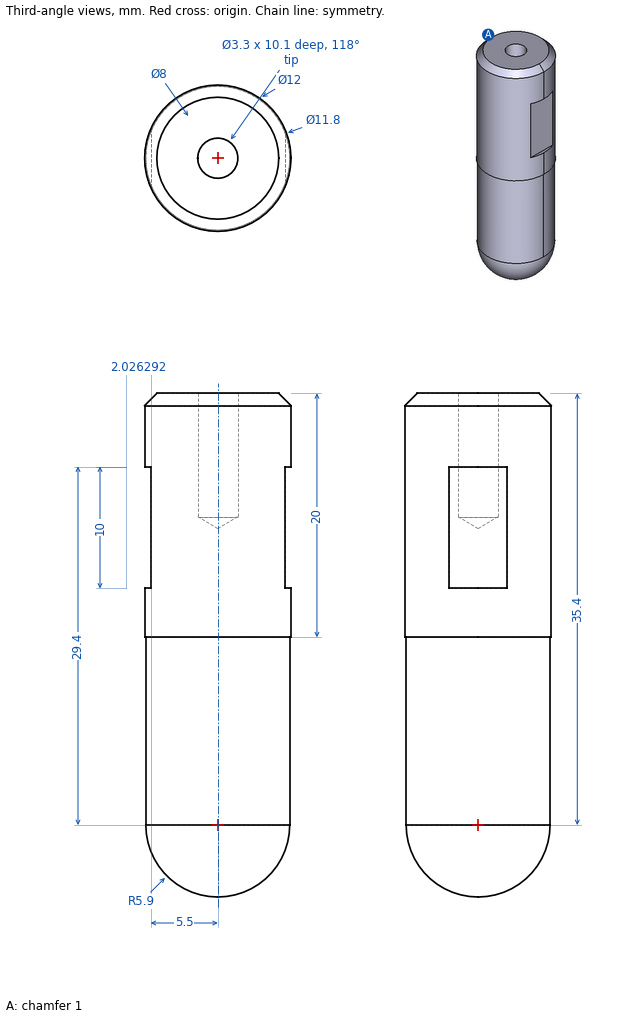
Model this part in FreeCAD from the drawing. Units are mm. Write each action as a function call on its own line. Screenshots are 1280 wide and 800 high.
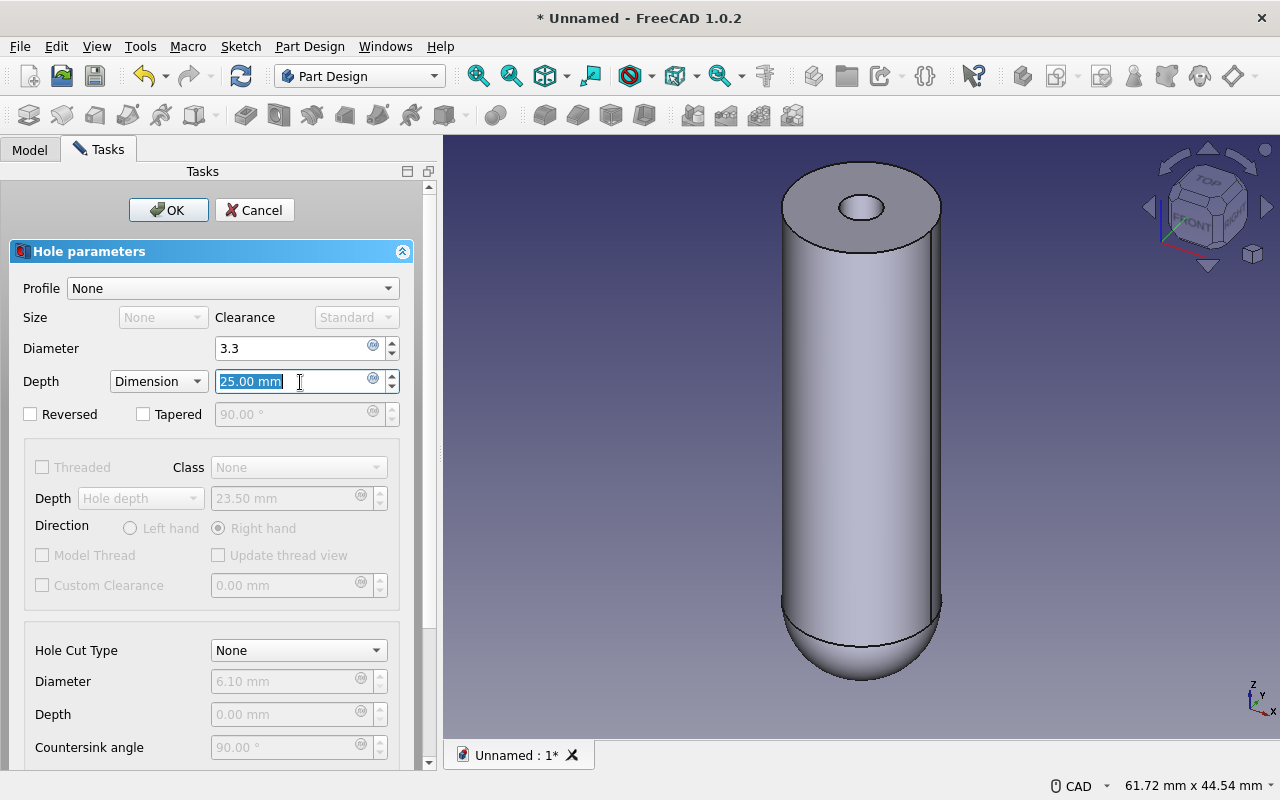
text(10.1)
key(Tab)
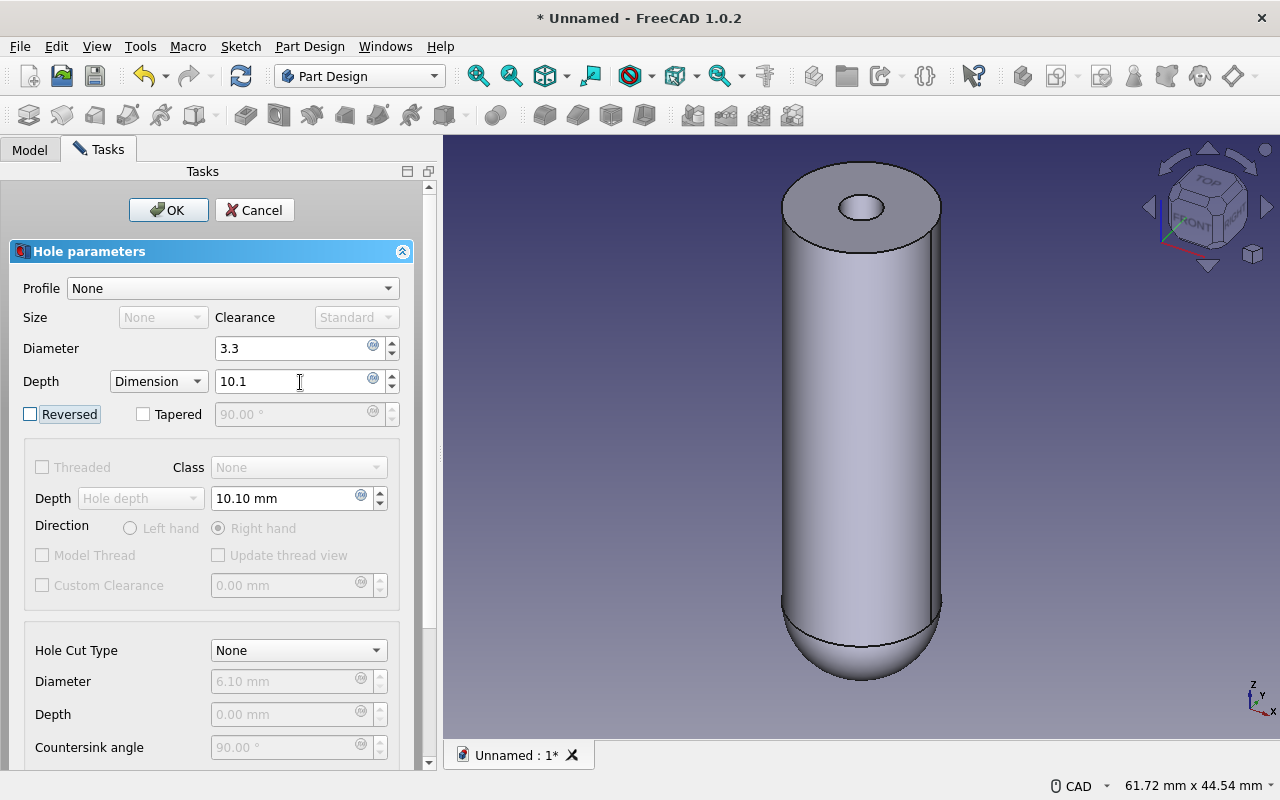
click(169, 210)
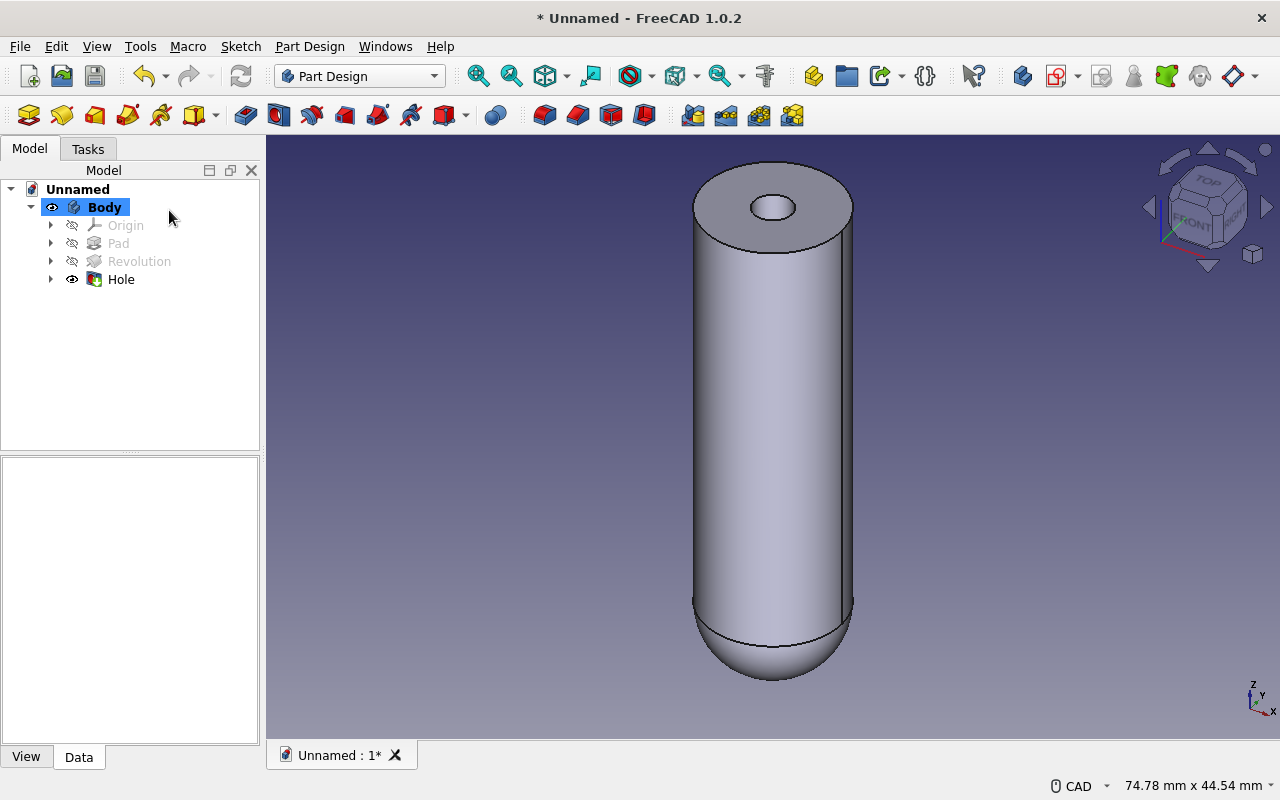
click(824, 208)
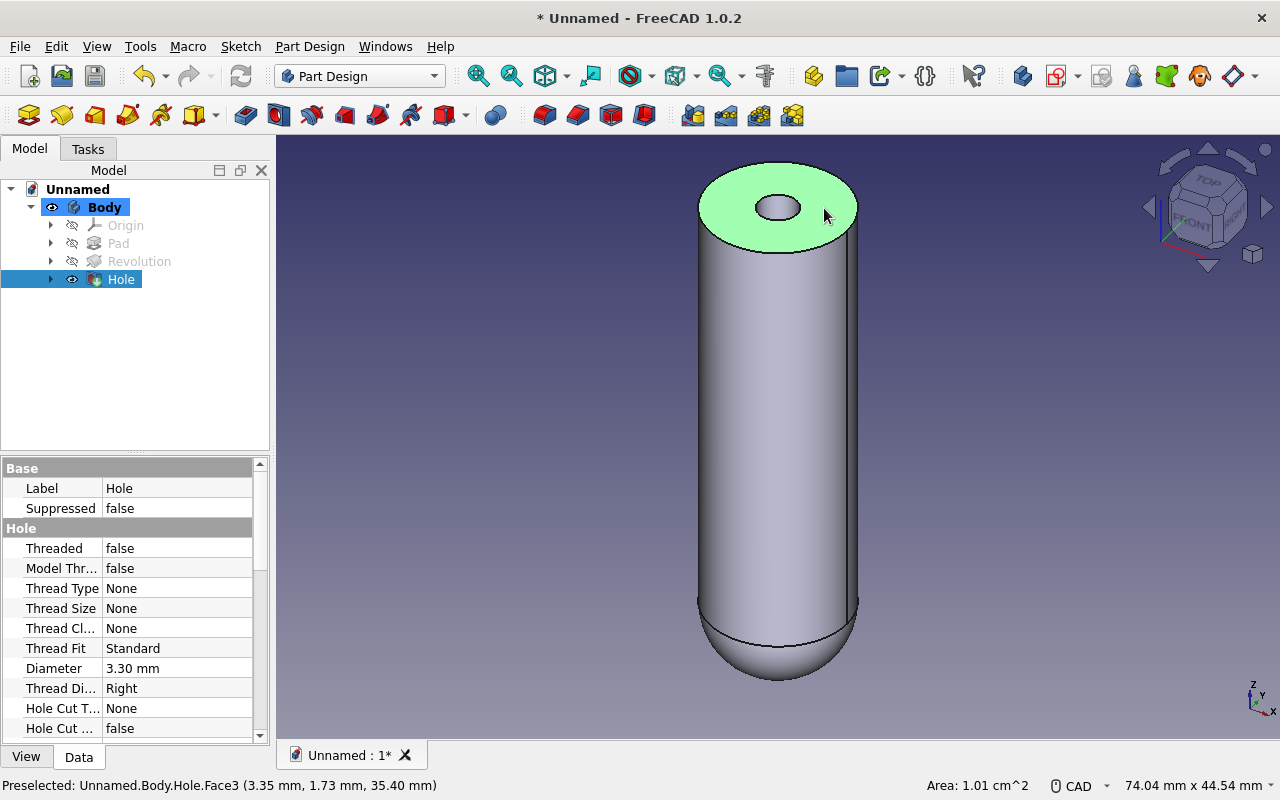
click(1056, 76)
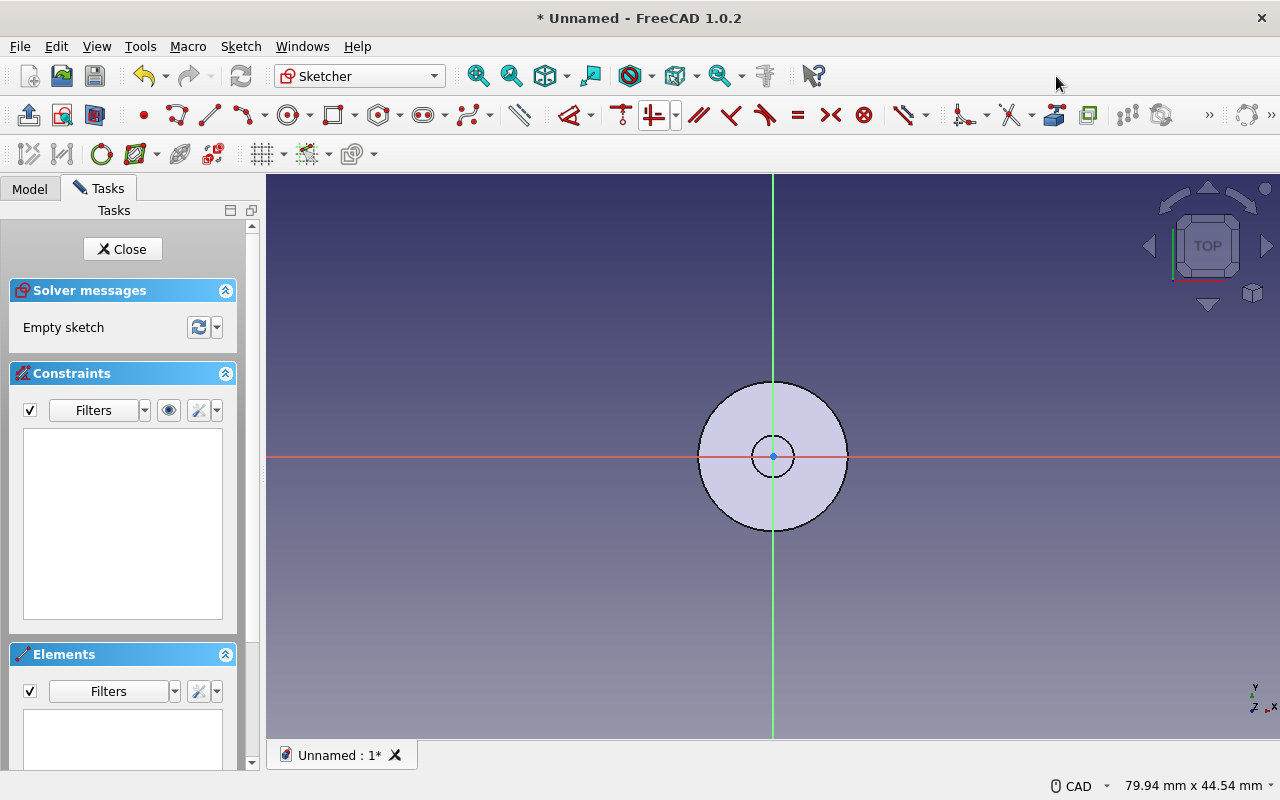
scroll(829, 456, up, 4)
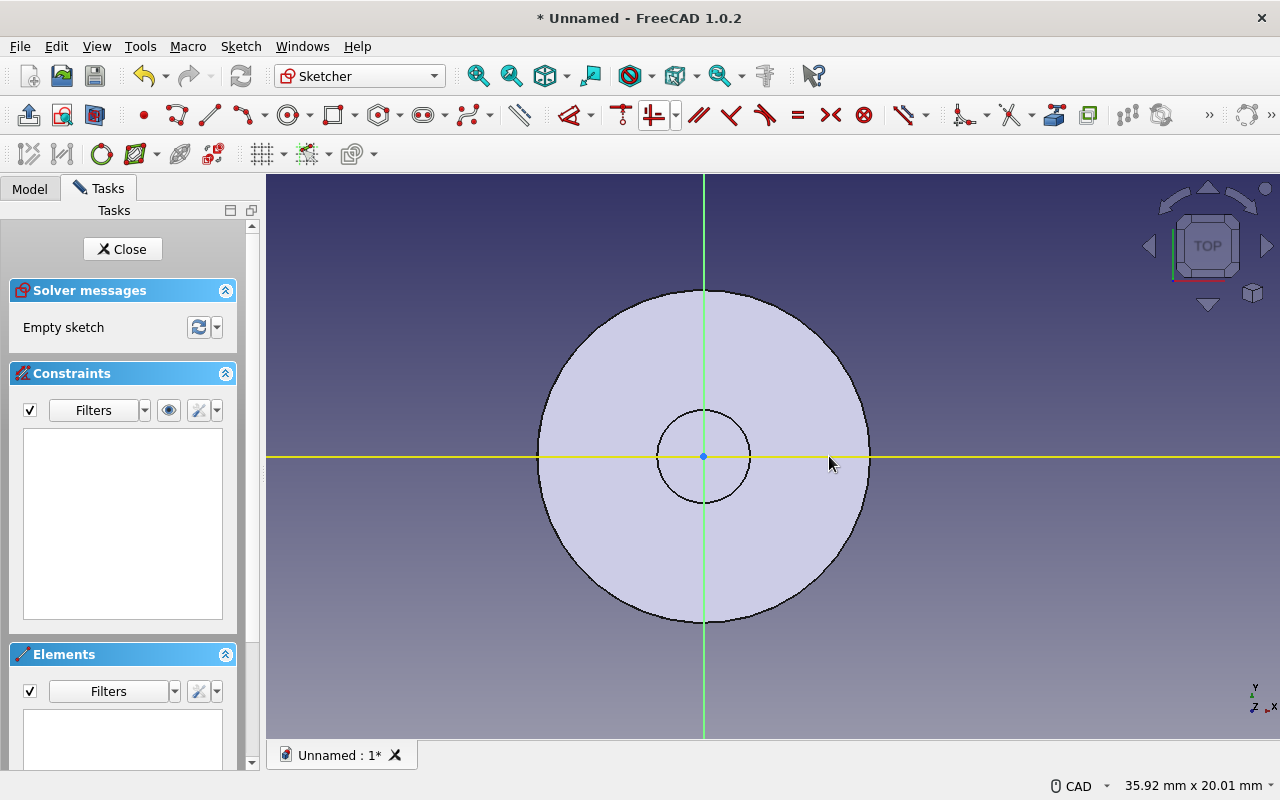
click(288, 116)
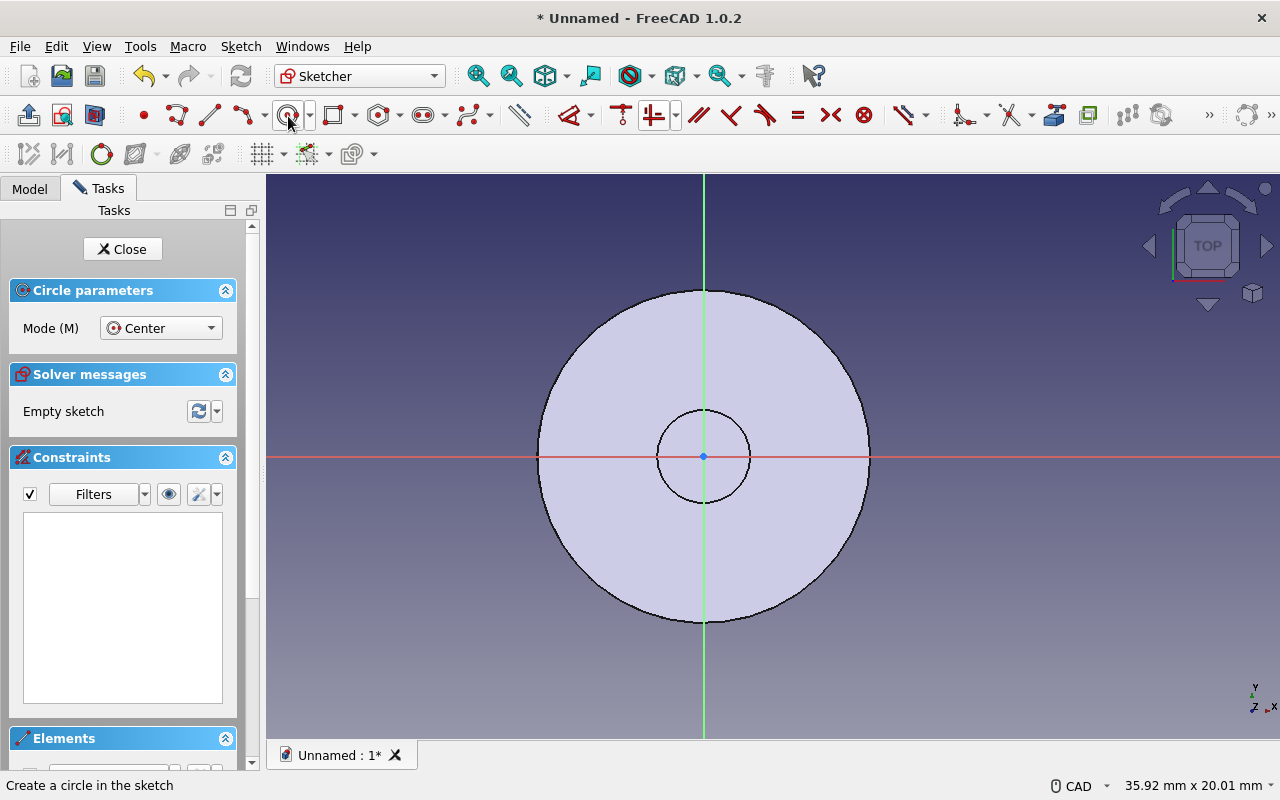
click(704, 456)
click(823, 337)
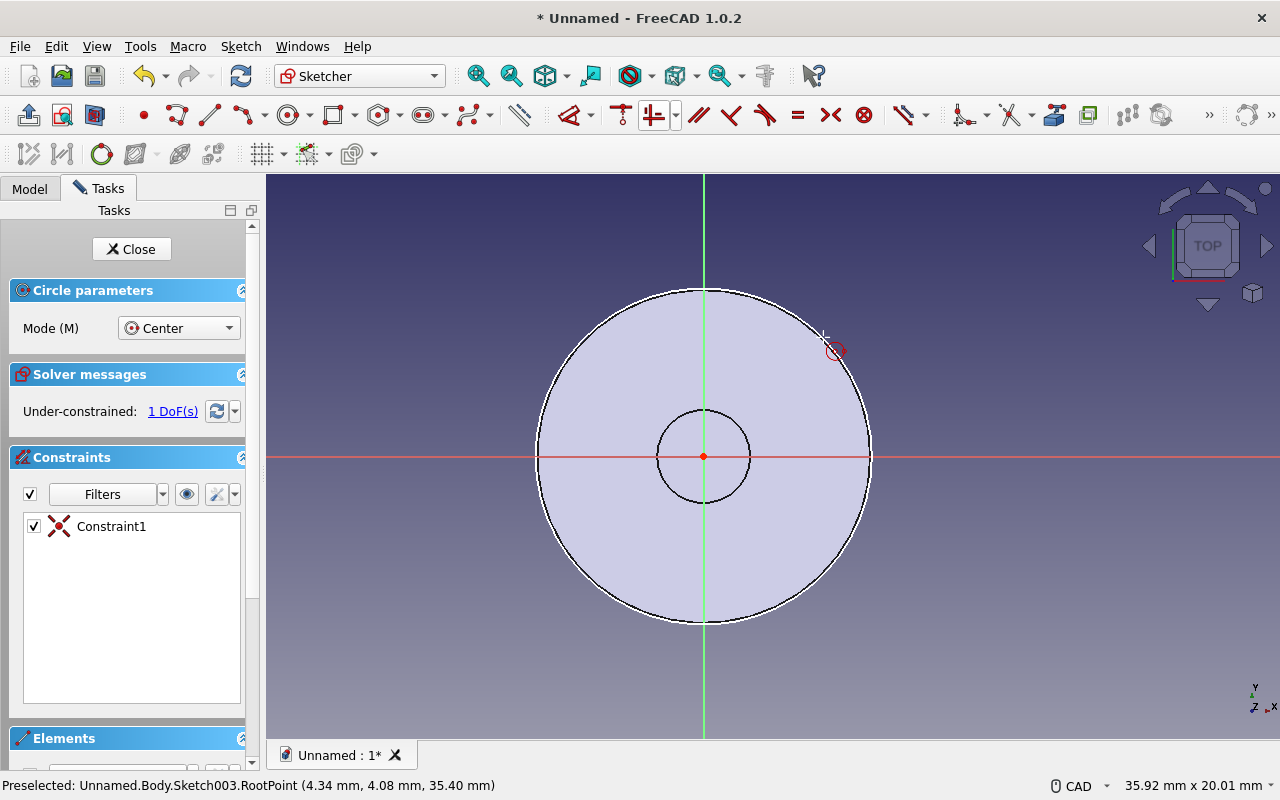
click(704, 456)
click(784, 377)
key(Escape)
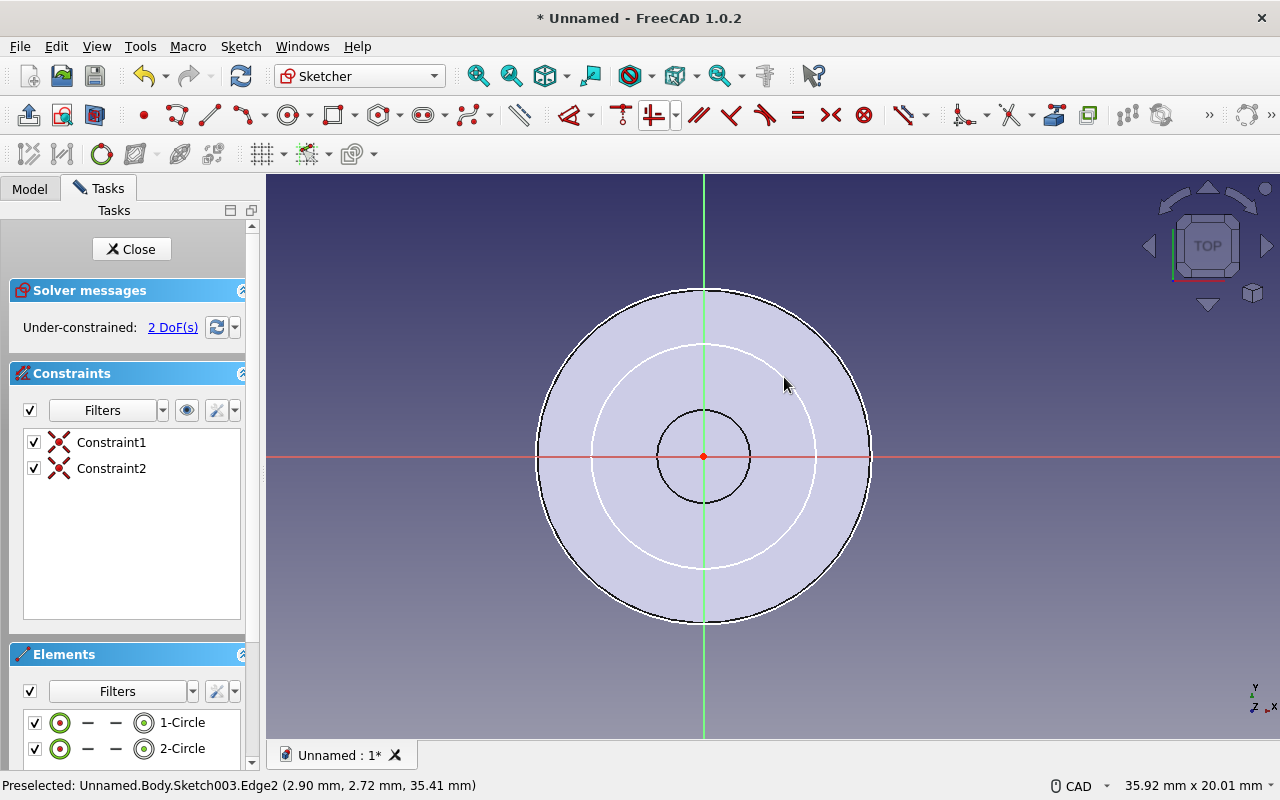
click(568, 116)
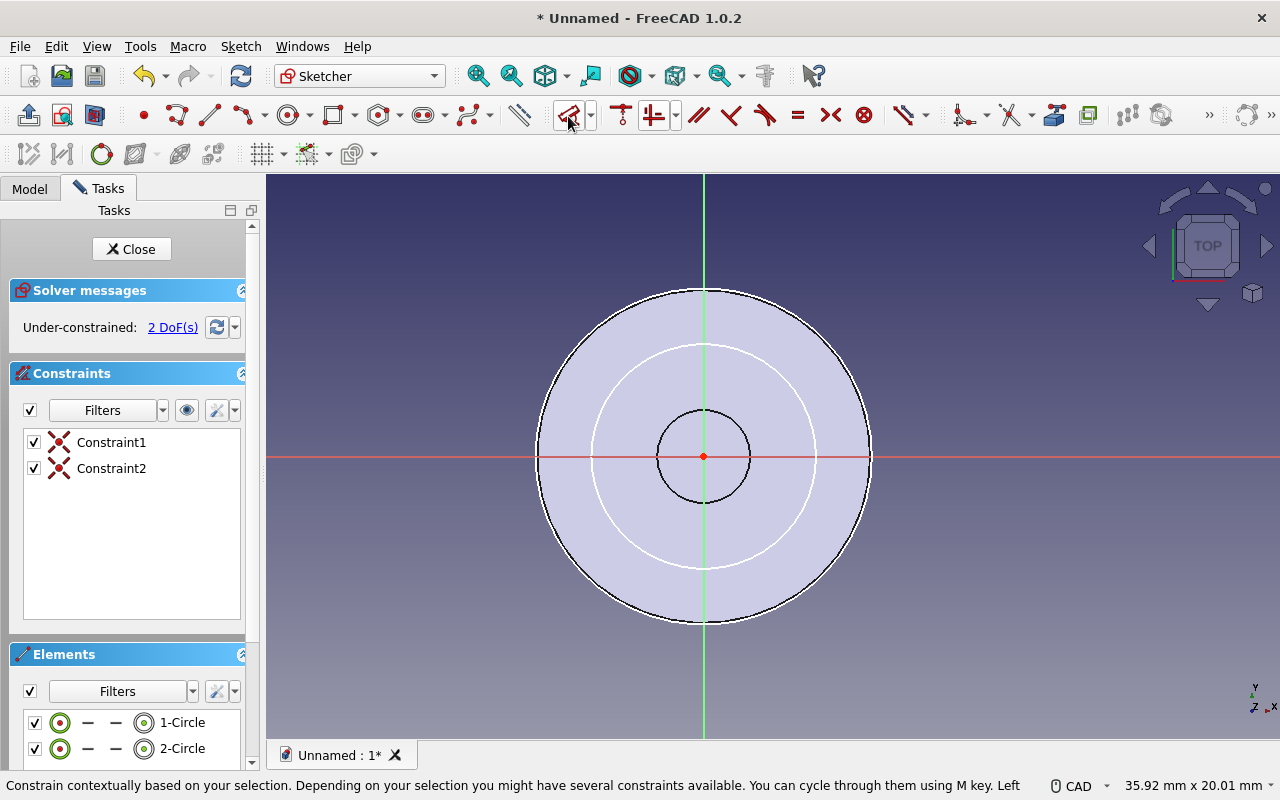
click(822, 337)
click(845, 314)